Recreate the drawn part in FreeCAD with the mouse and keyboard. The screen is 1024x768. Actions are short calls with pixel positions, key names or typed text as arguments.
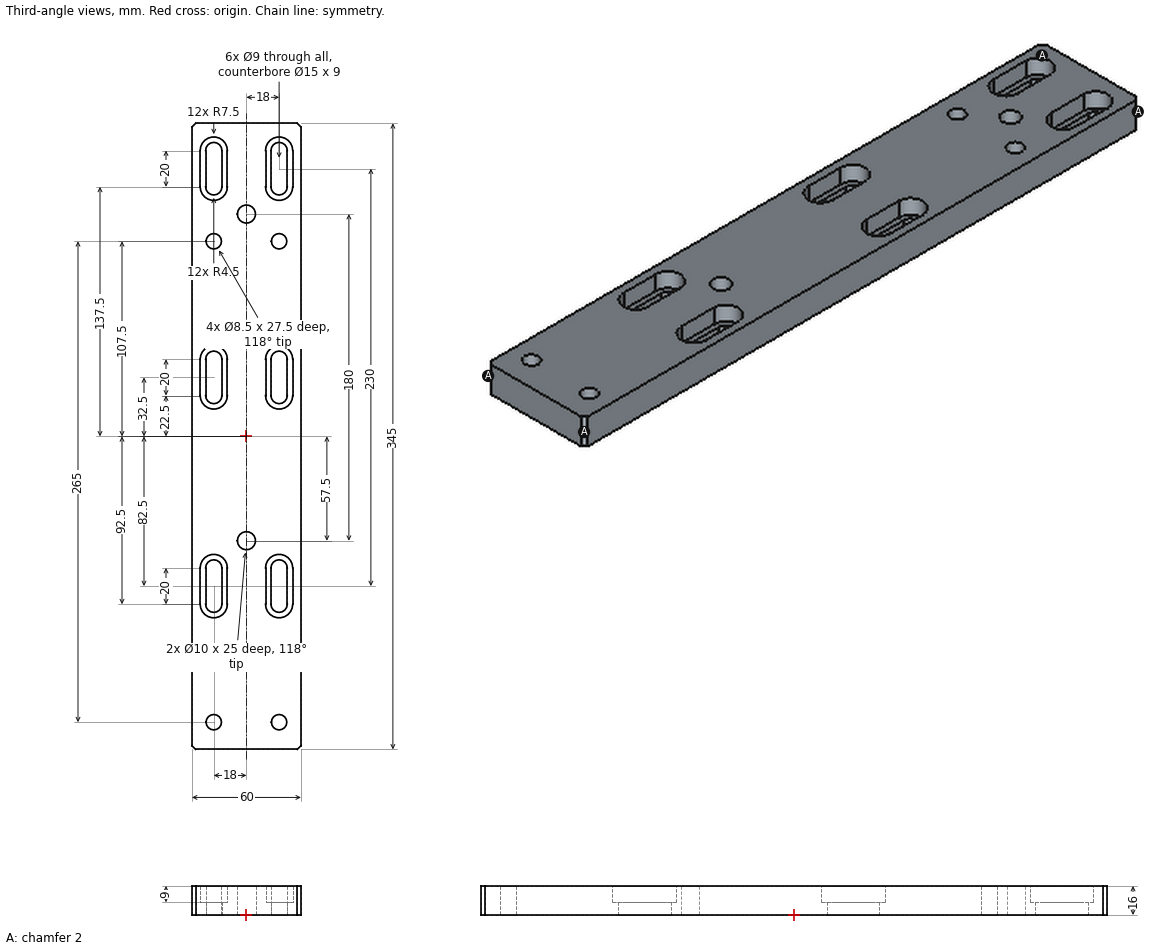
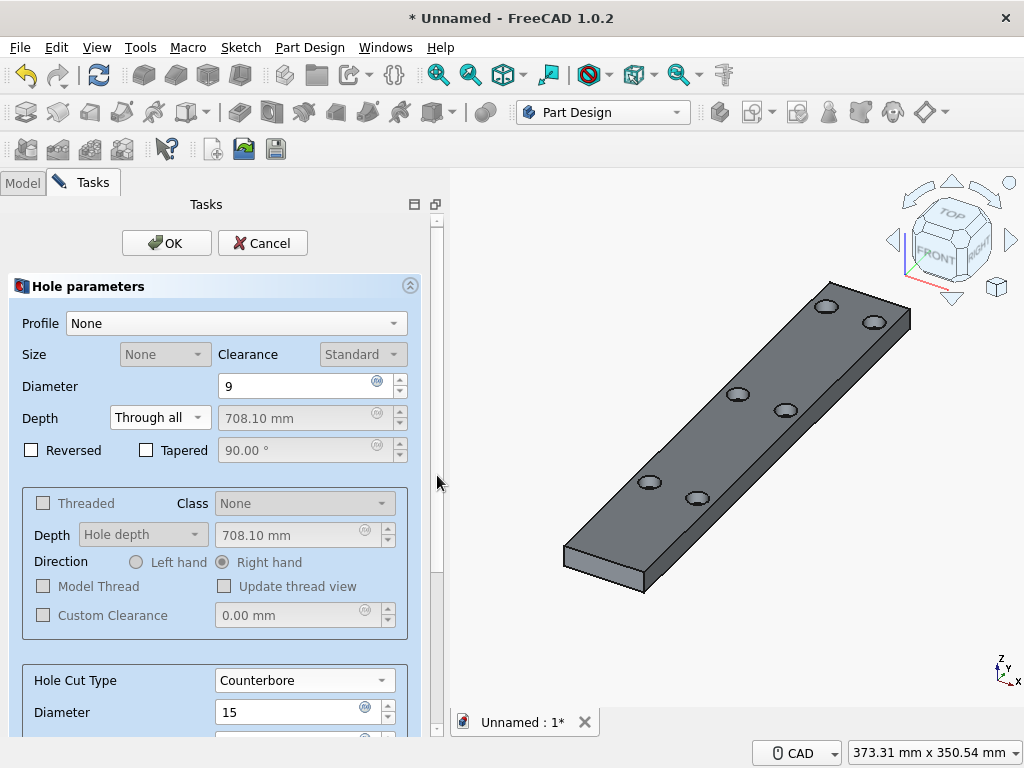
click(167, 243)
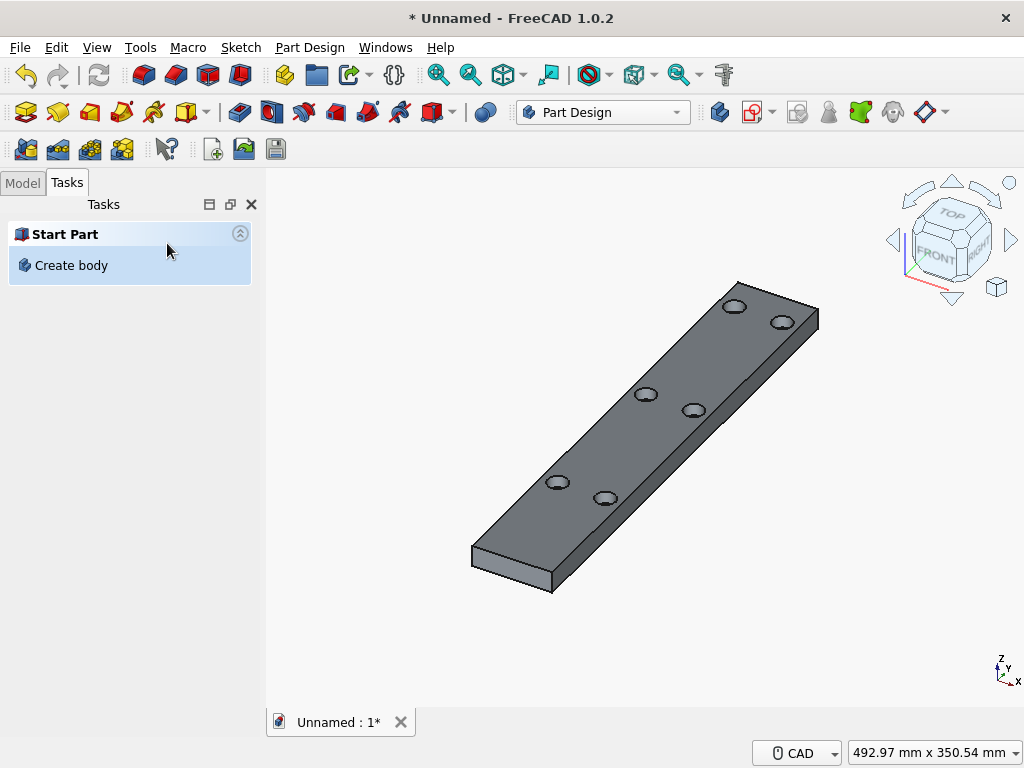
click(552, 581)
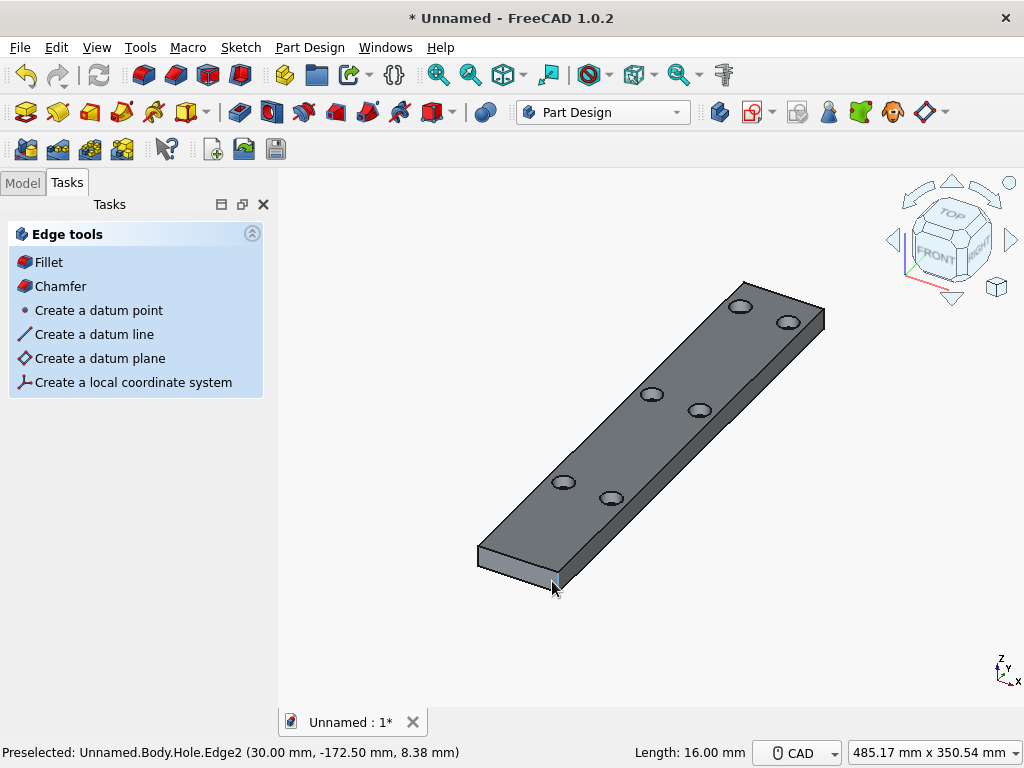
key(0)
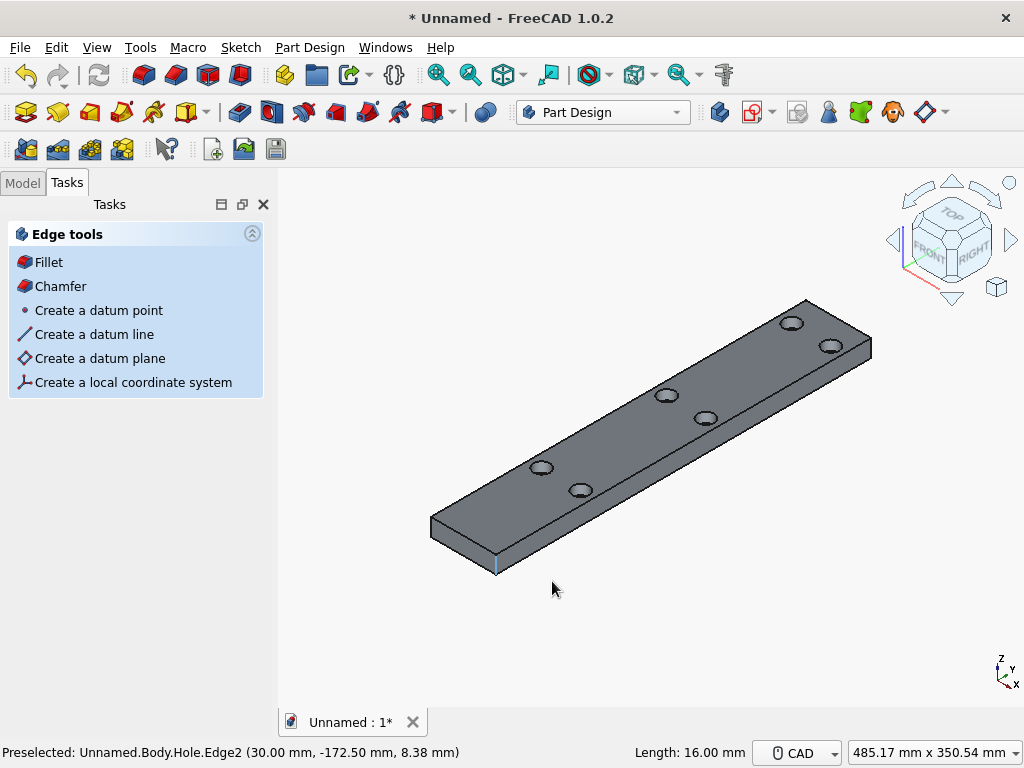
key(2)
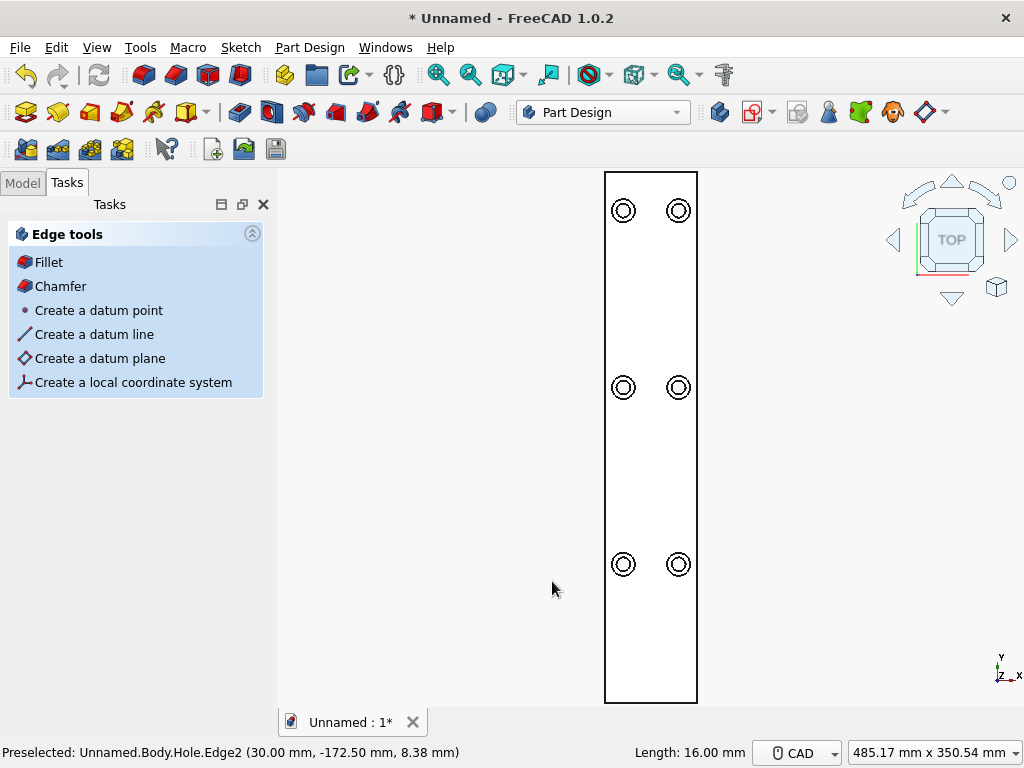
key(1)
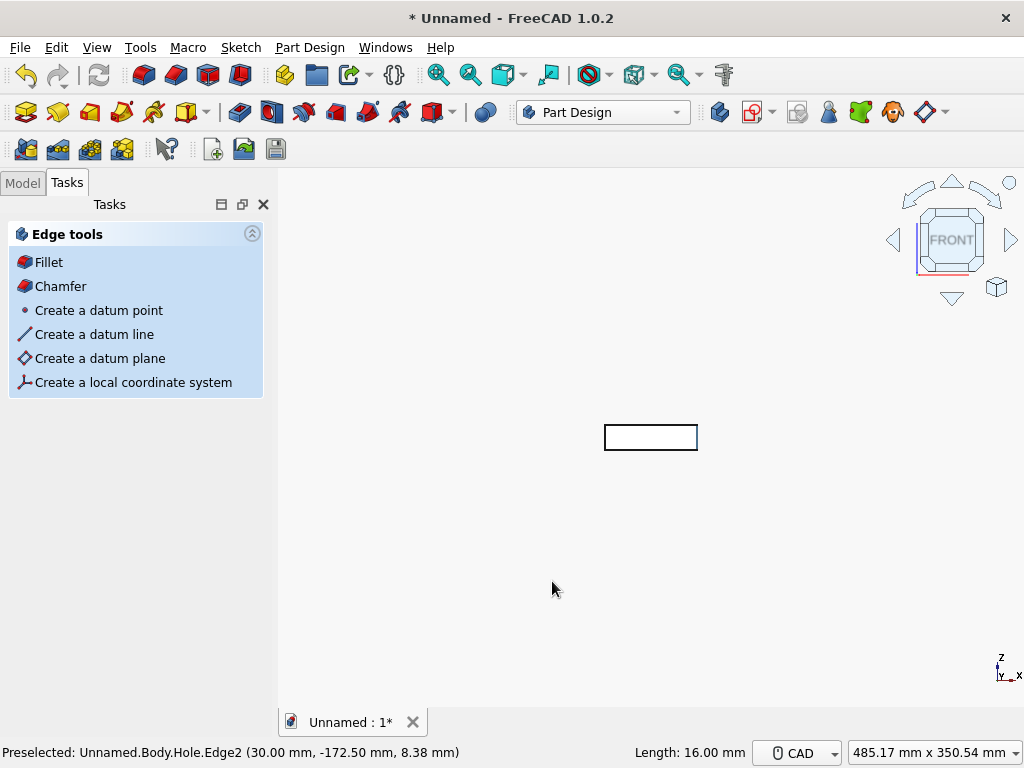
click(440, 76)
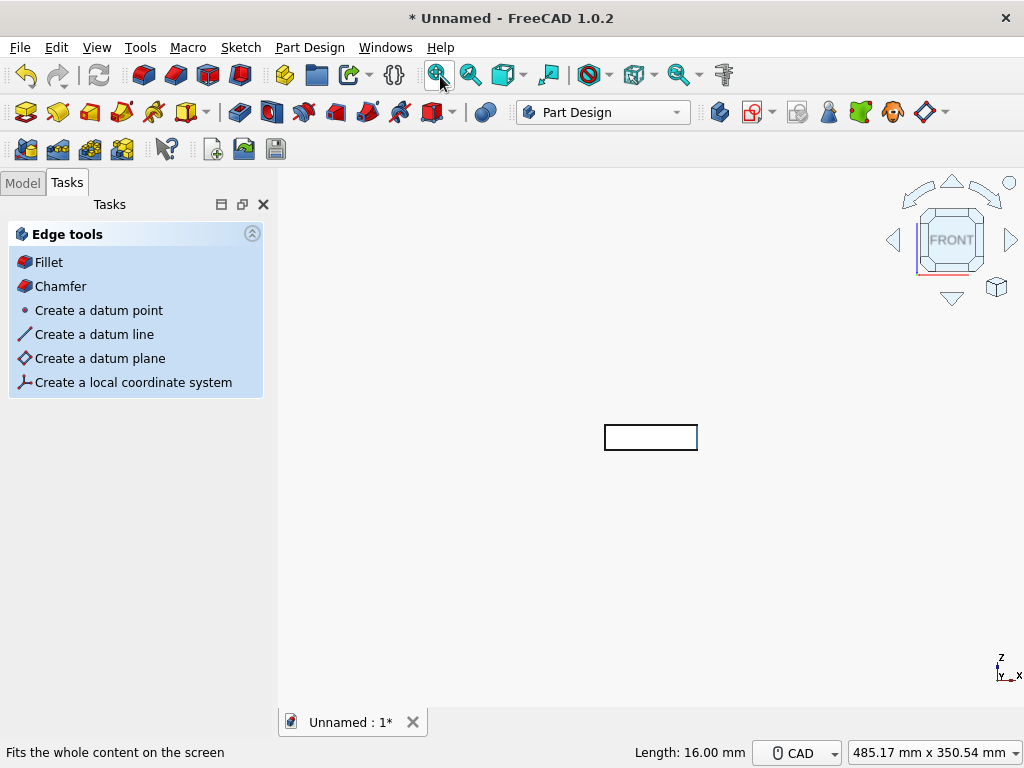
click(605, 437, ctrl)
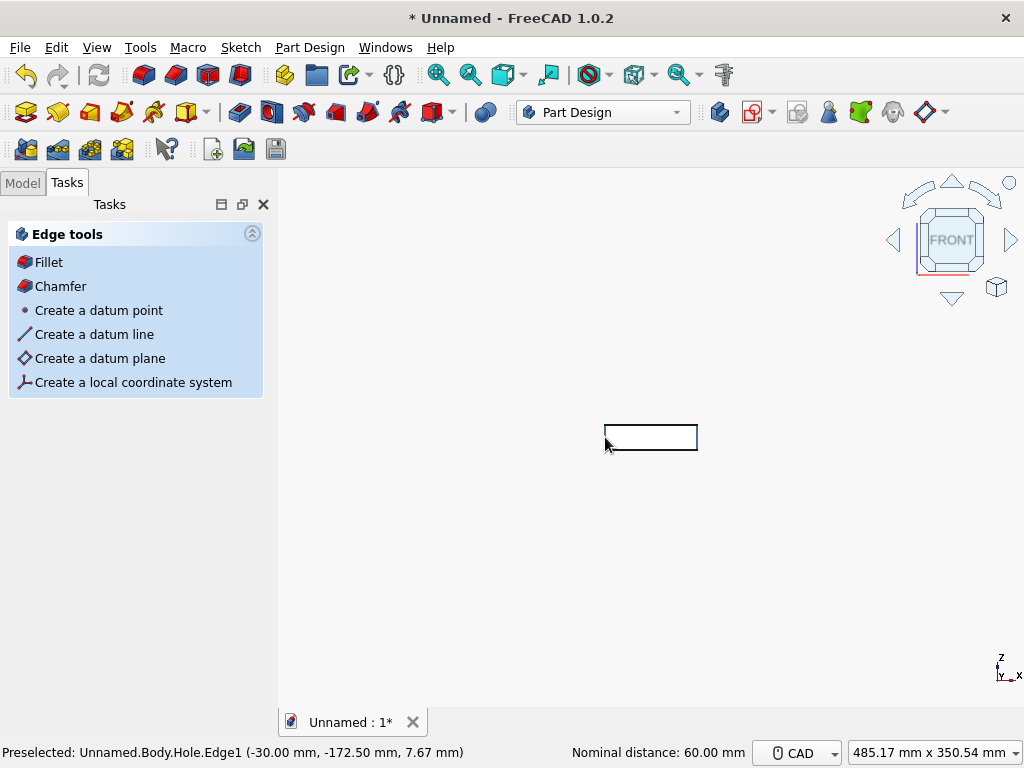
key(3)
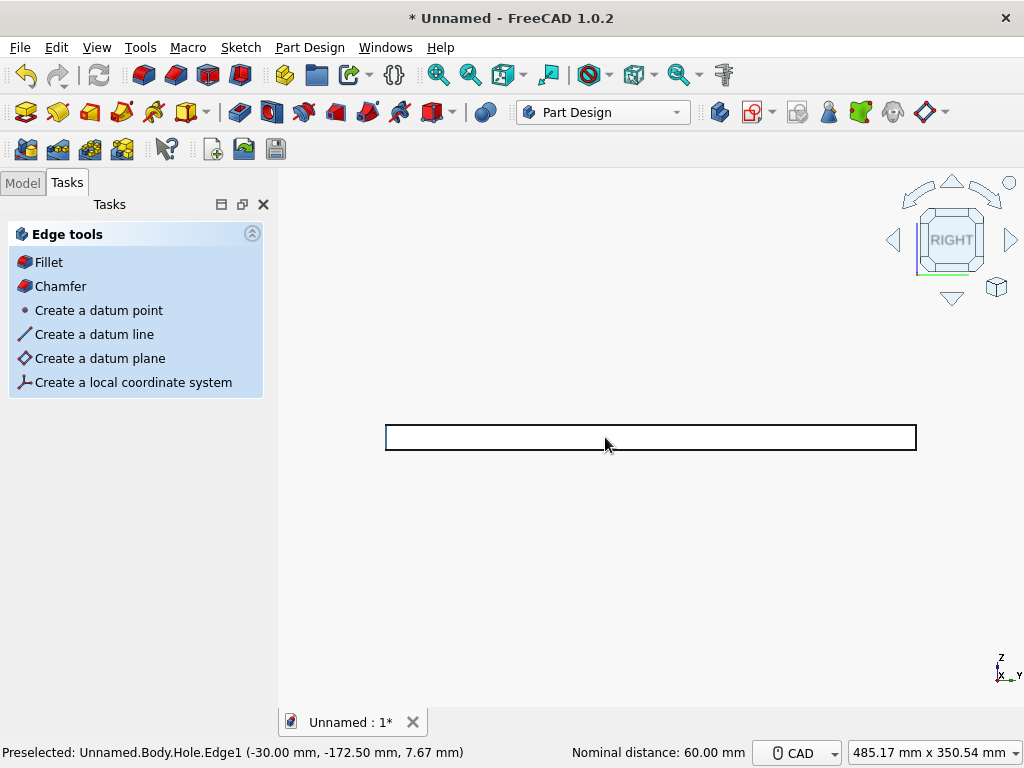
click(916, 436, ctrl)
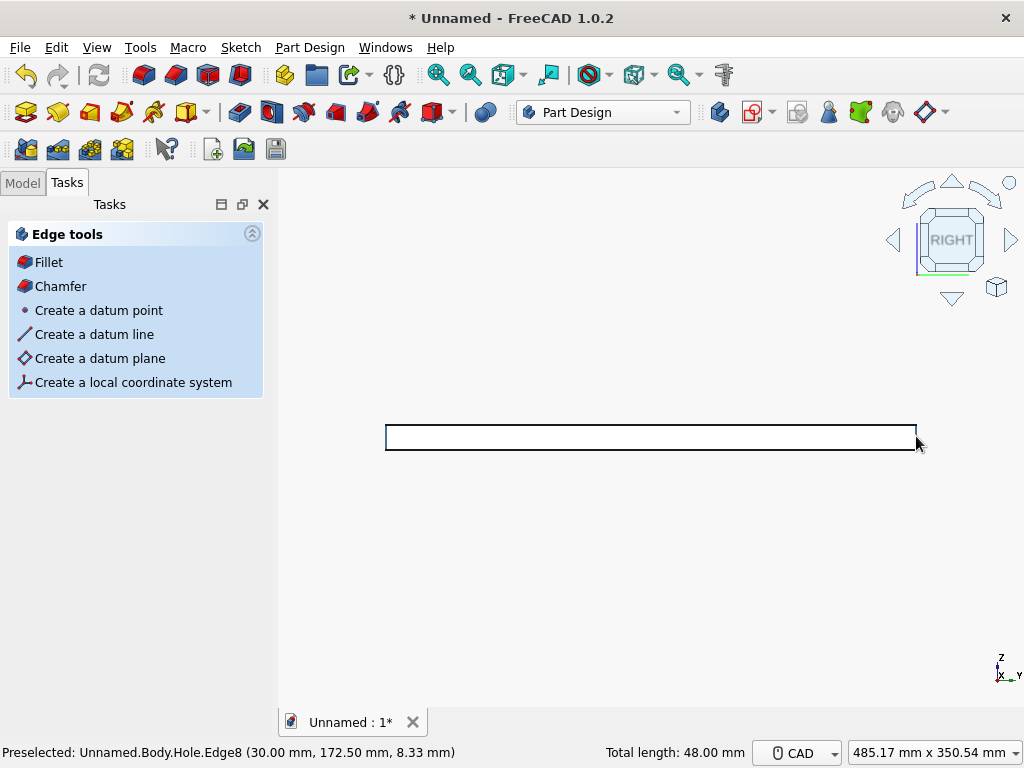
key(5)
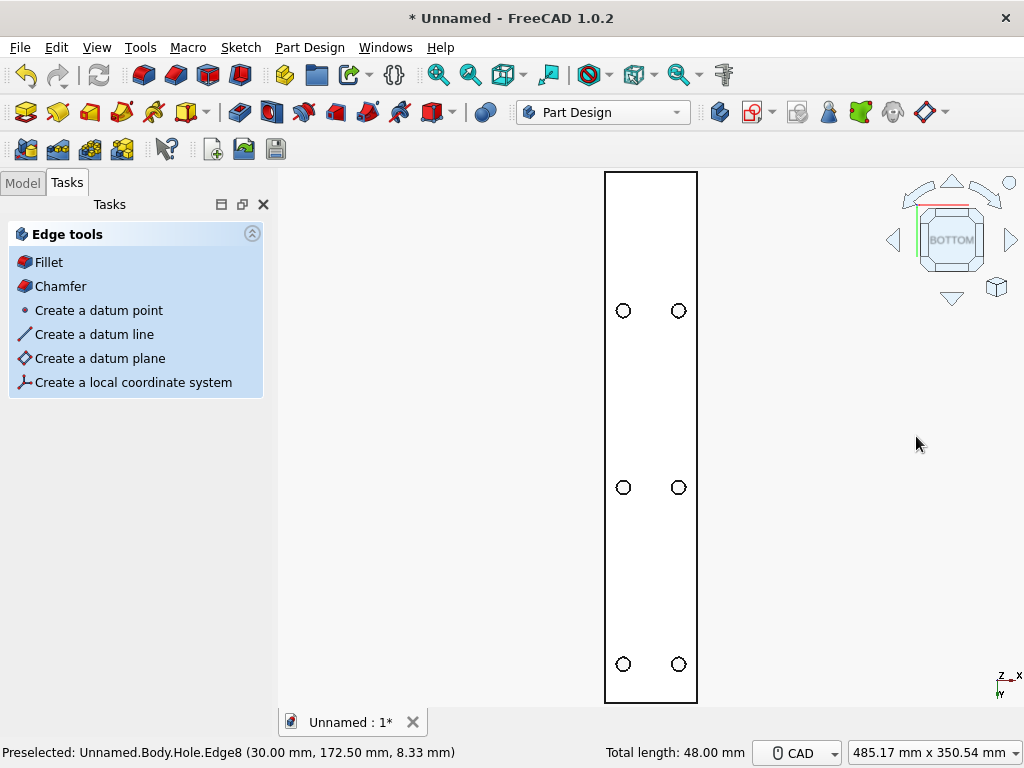
key(4)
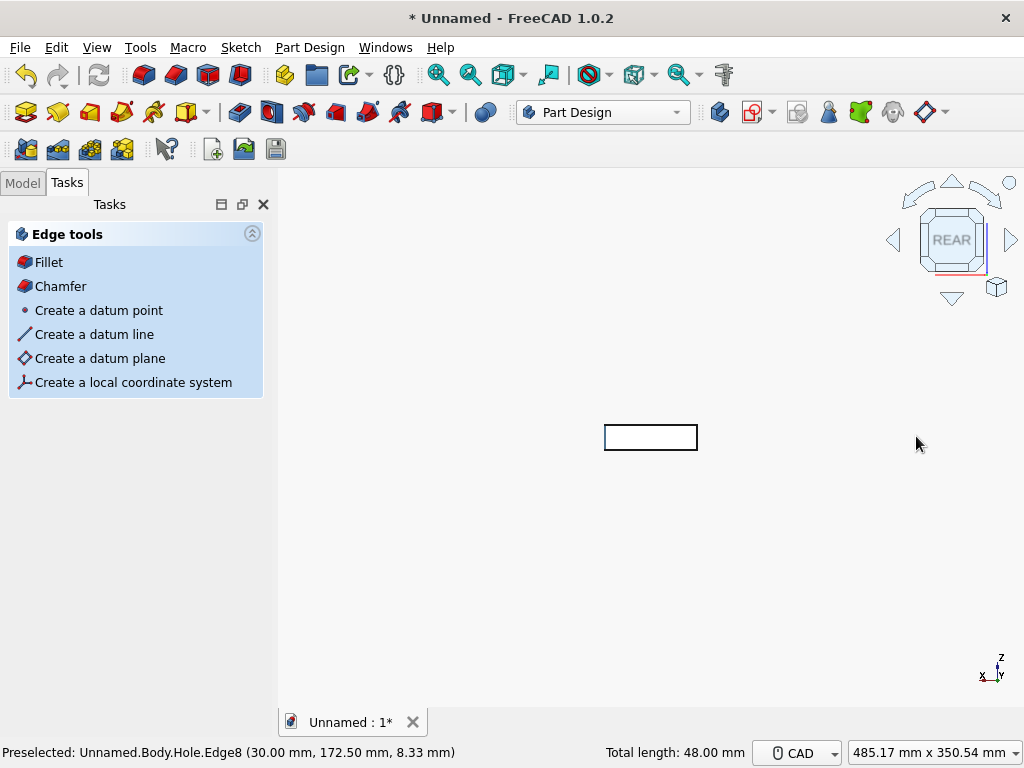
key(v)
key(f)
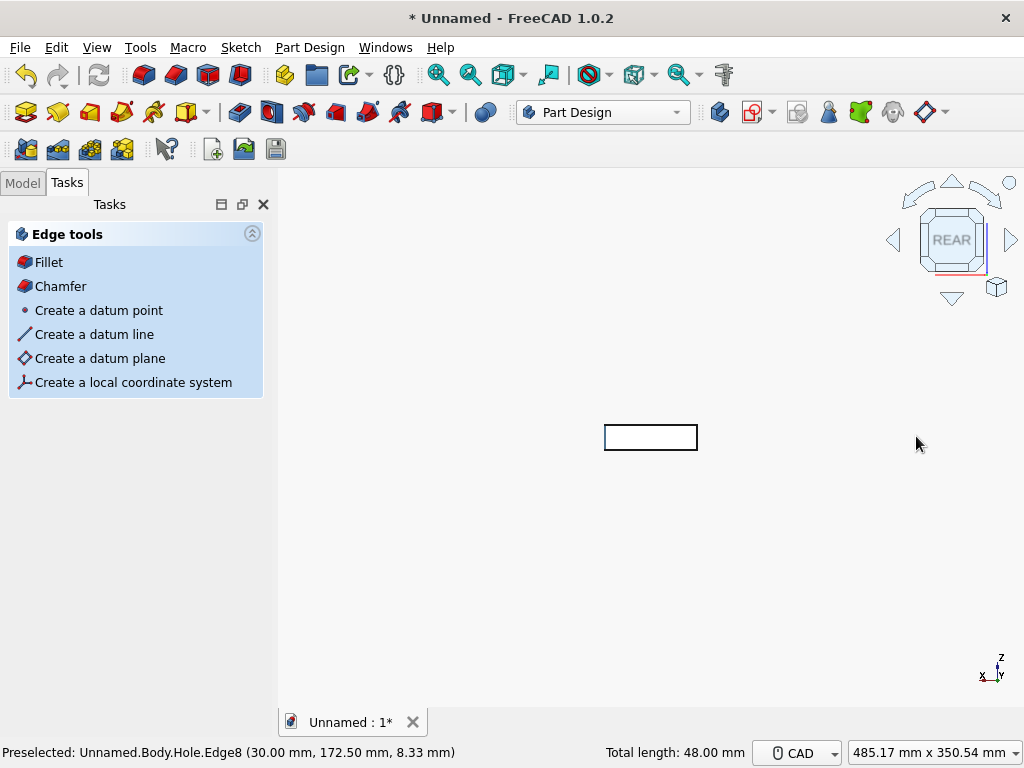
click(697, 437, ctrl)